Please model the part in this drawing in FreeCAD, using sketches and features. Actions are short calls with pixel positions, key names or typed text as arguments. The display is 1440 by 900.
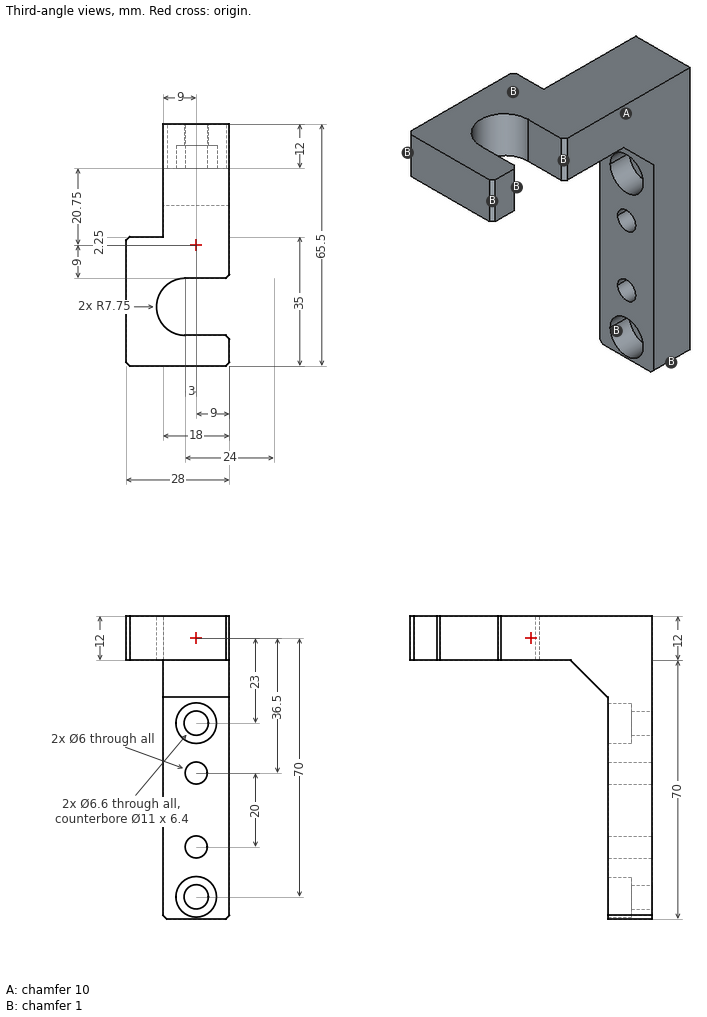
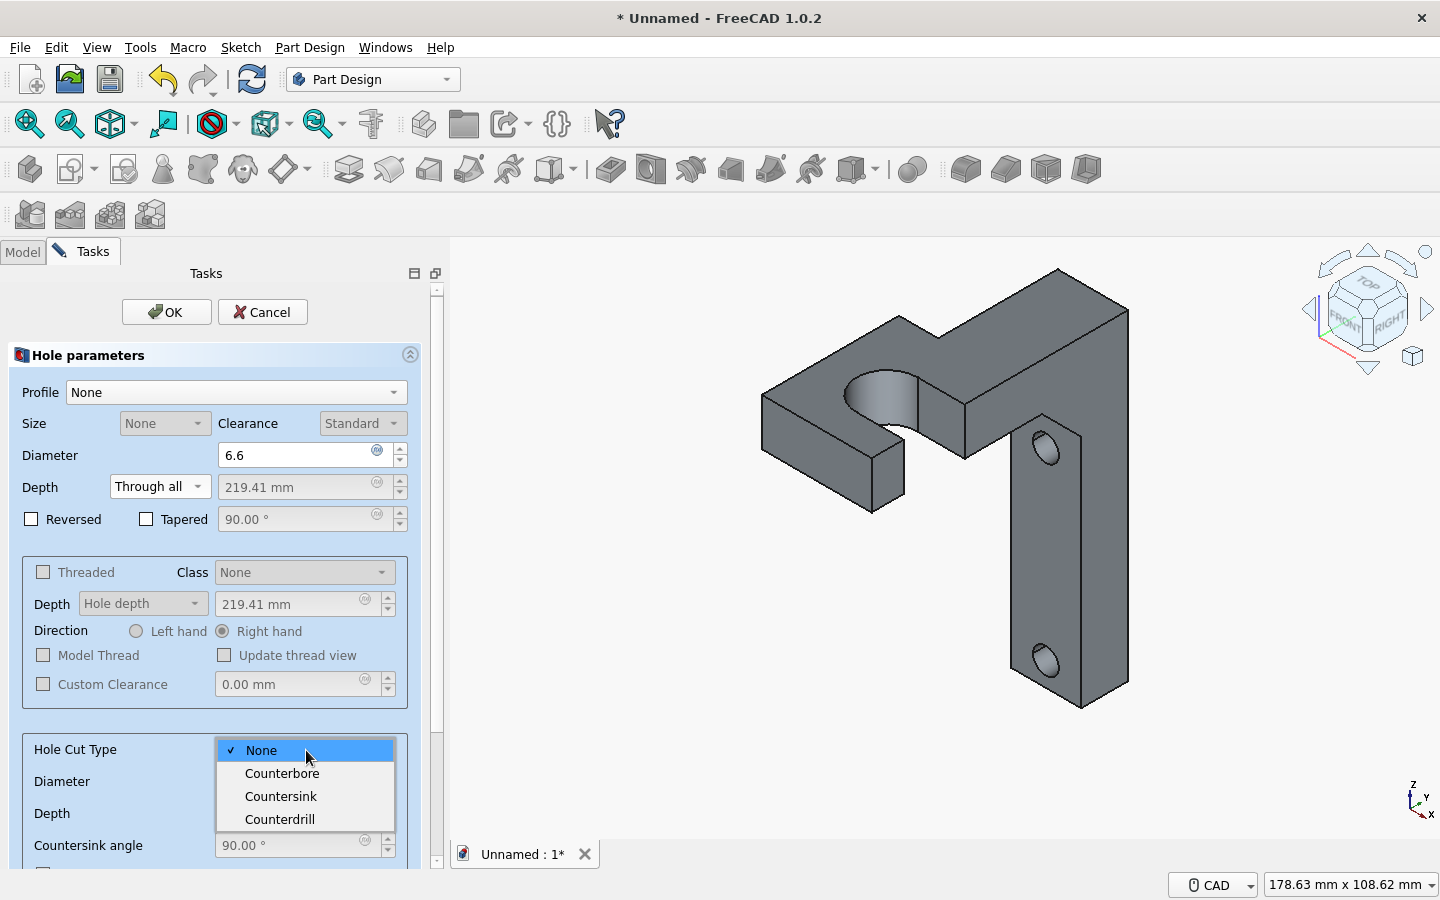
click(304, 774)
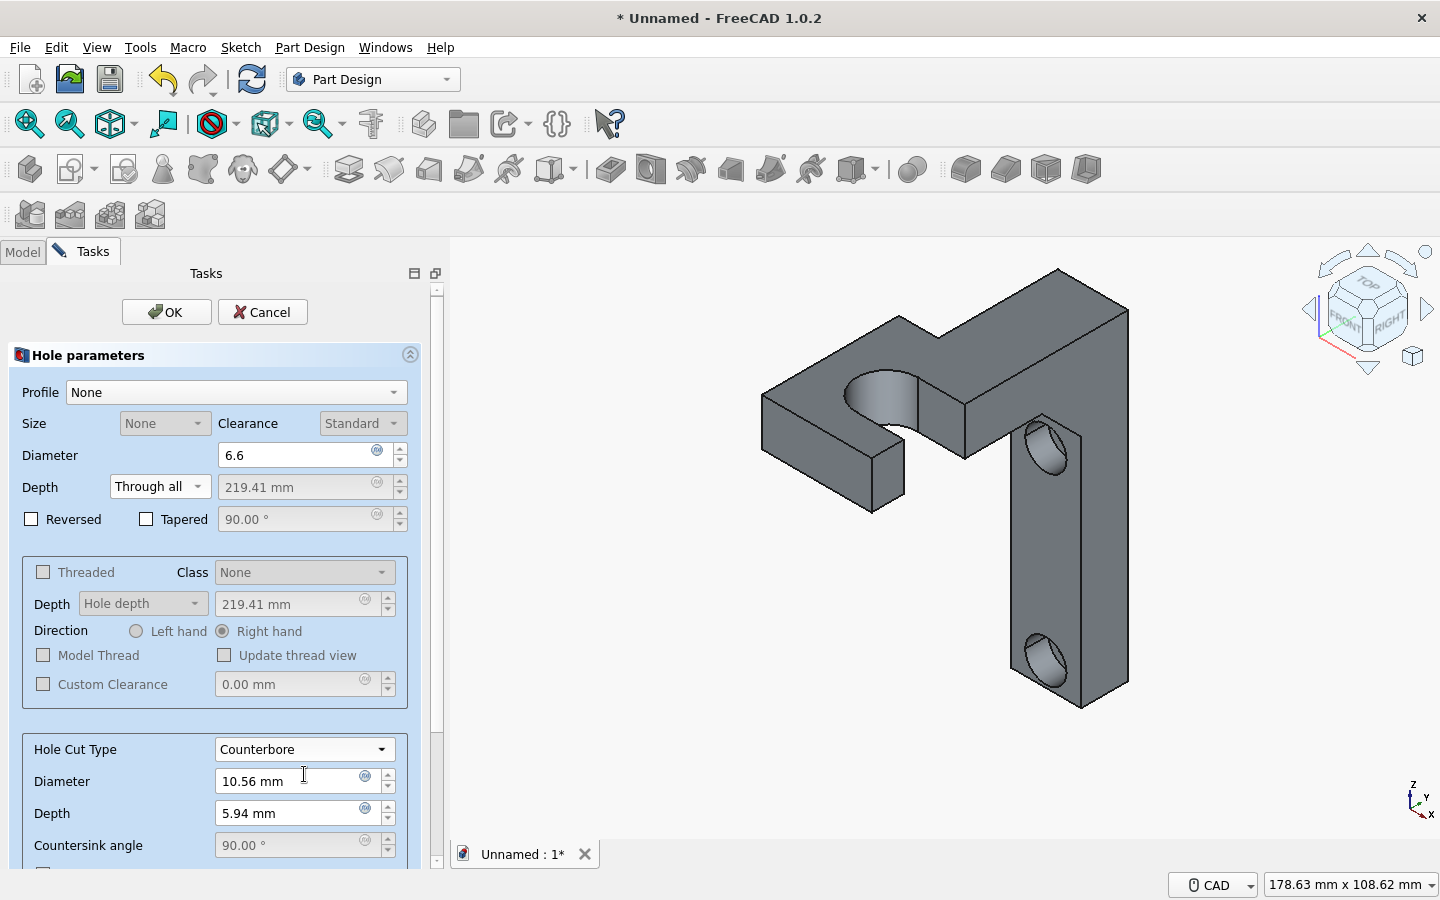
triple_click(298, 781)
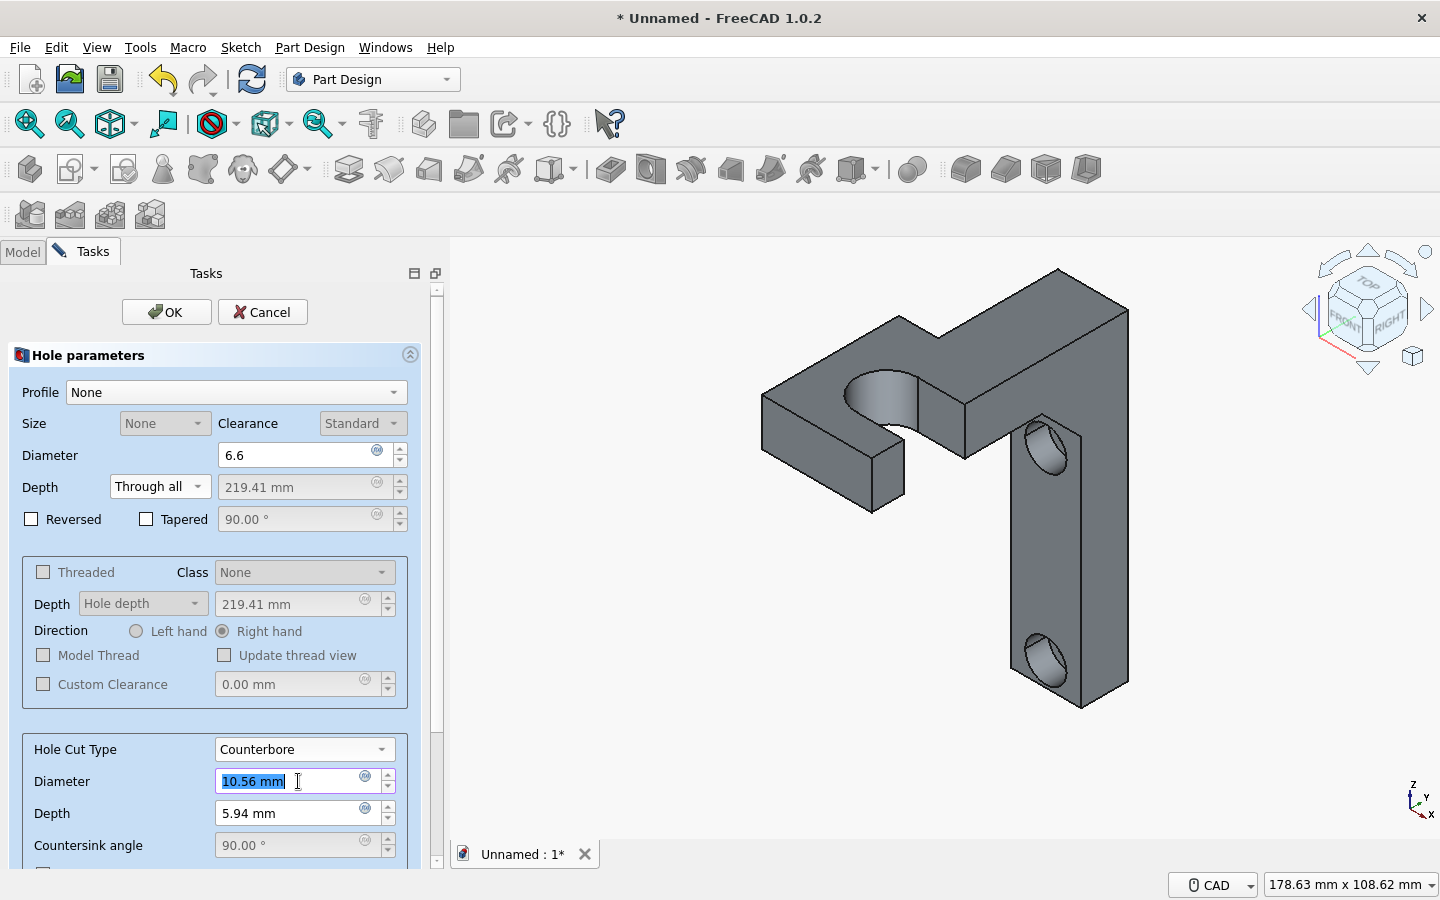
text(11)
key(Tab)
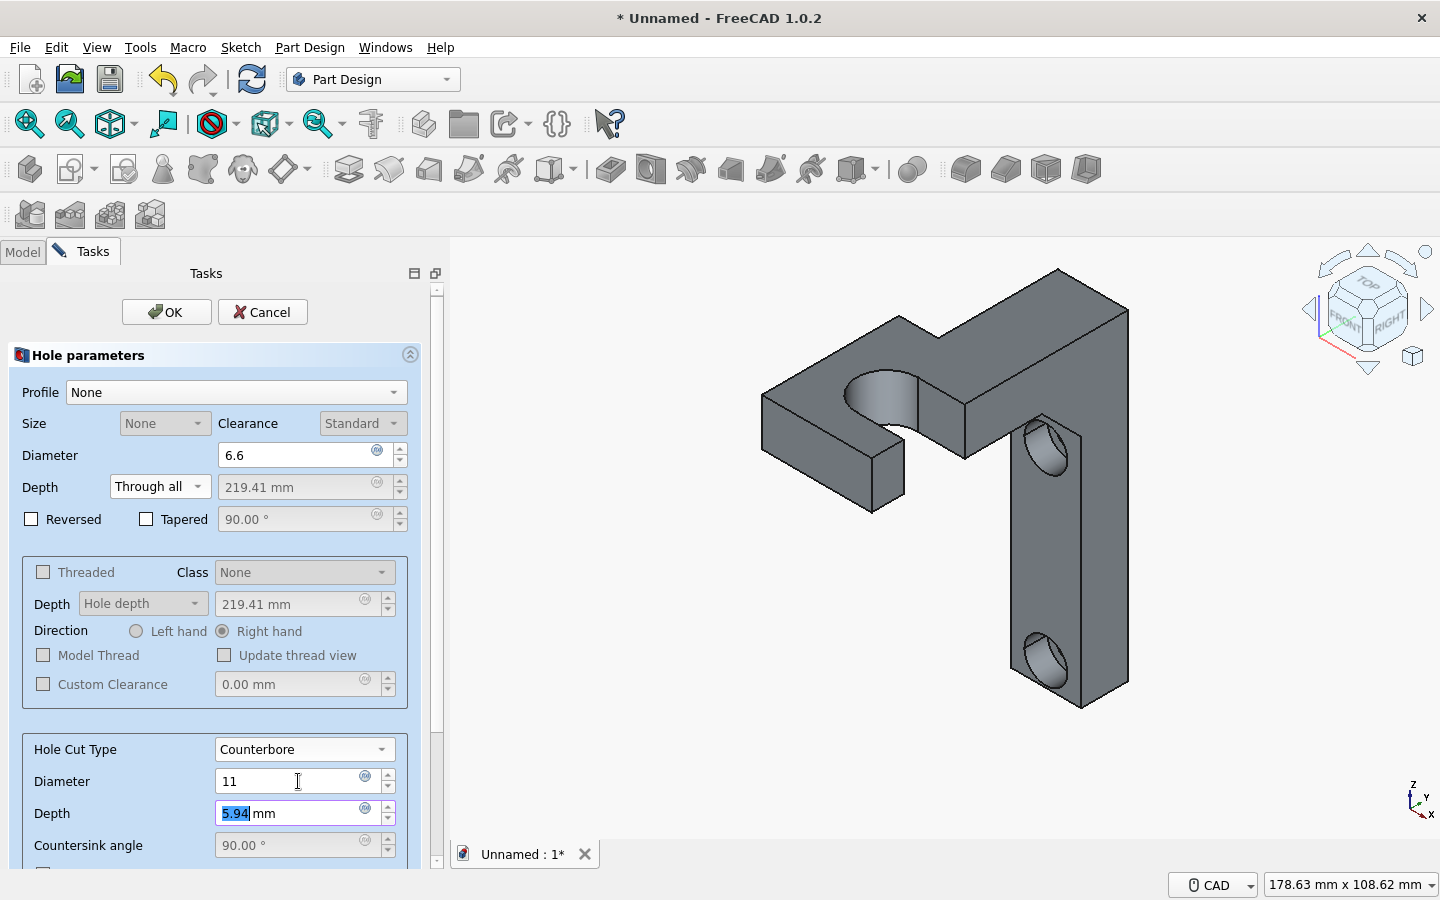
text(6.4)
key(Tab)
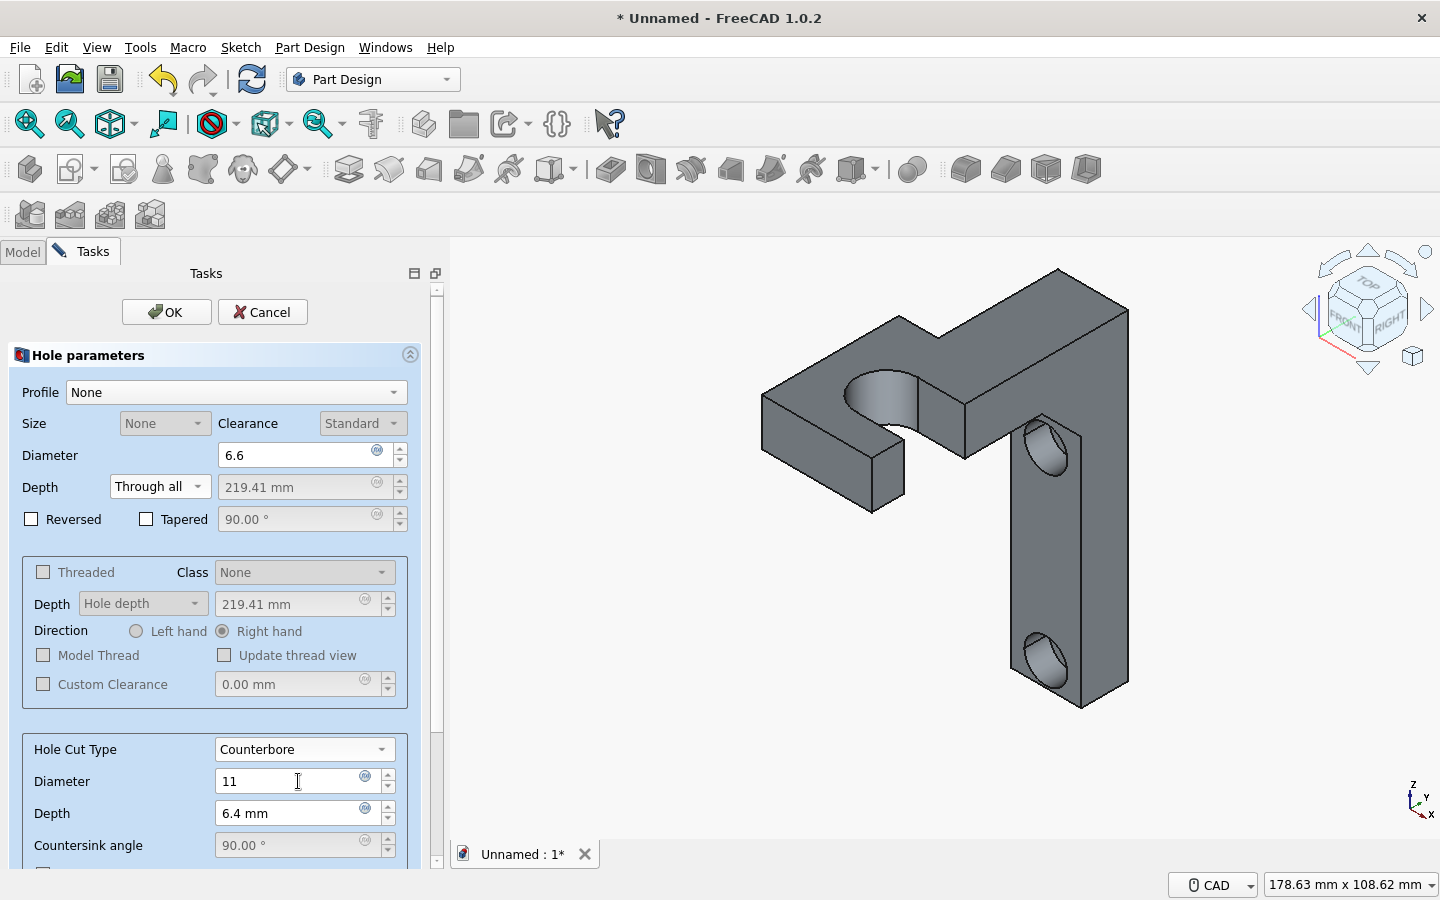
click(167, 312)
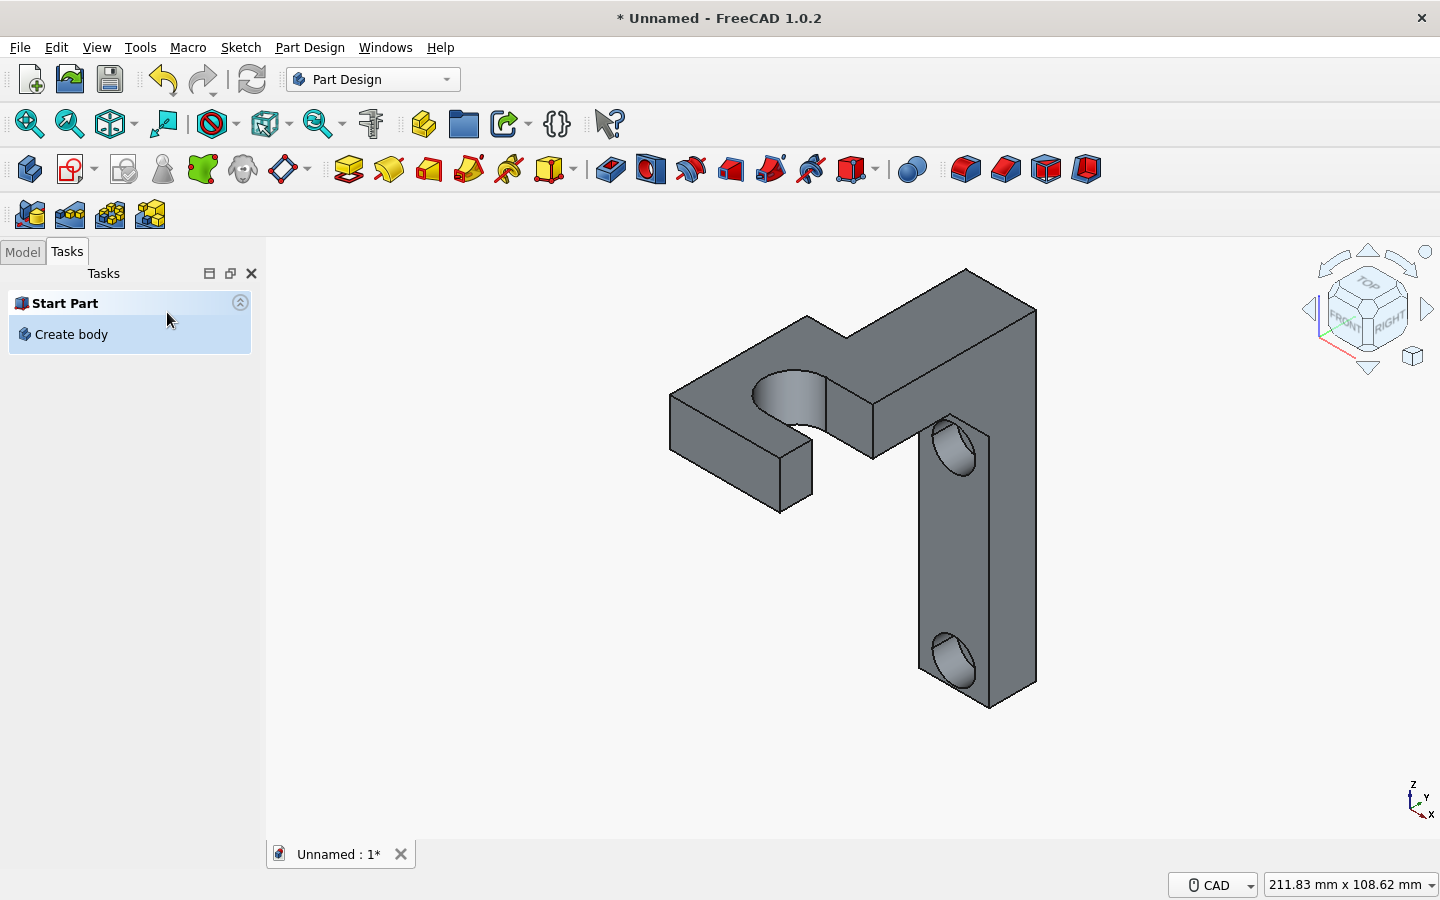
click(954, 551)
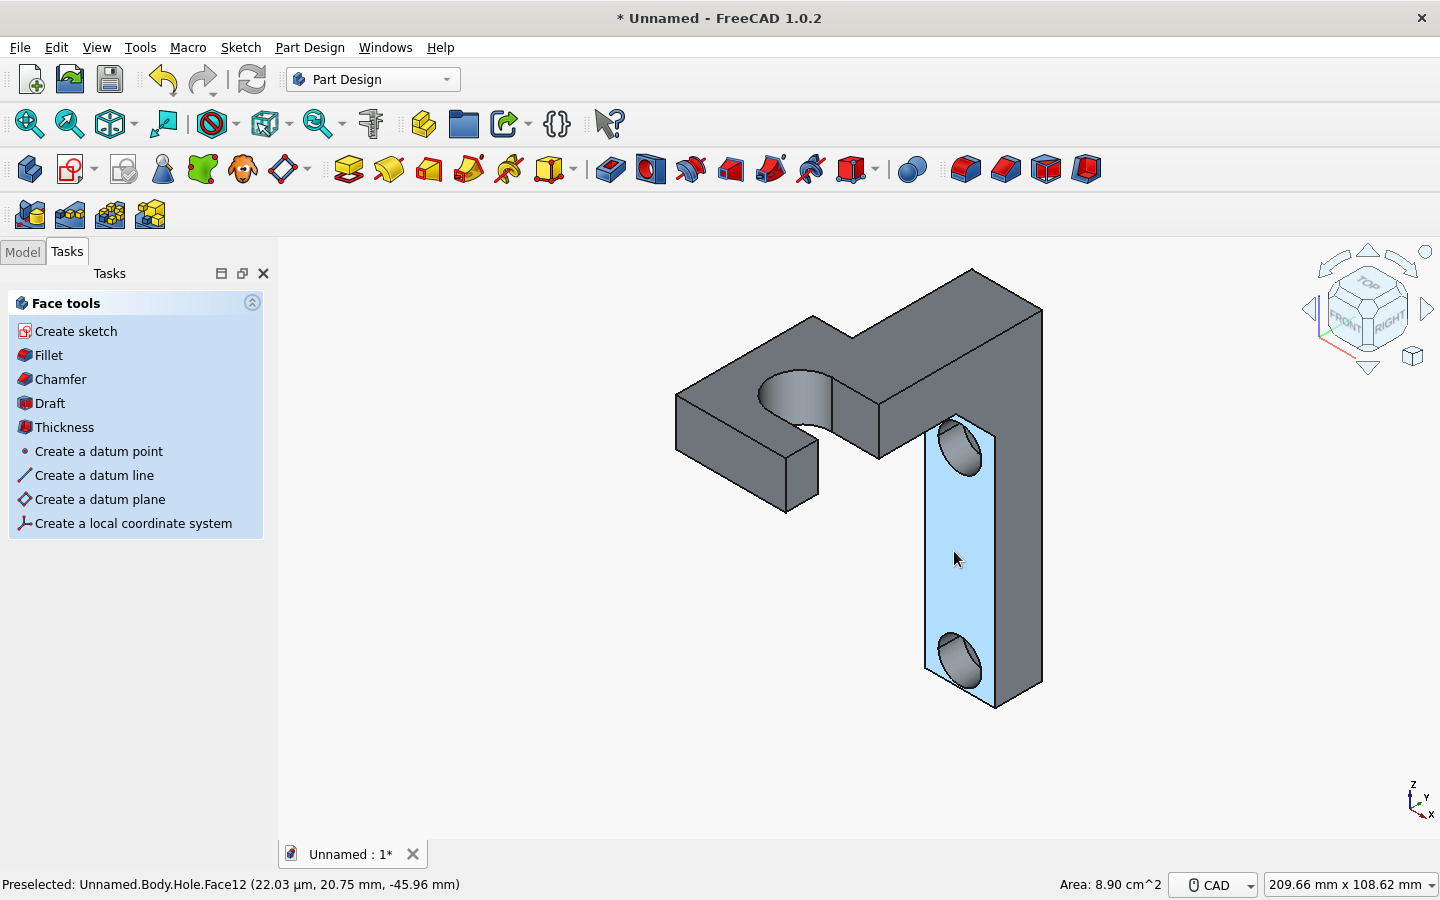
click(70, 170)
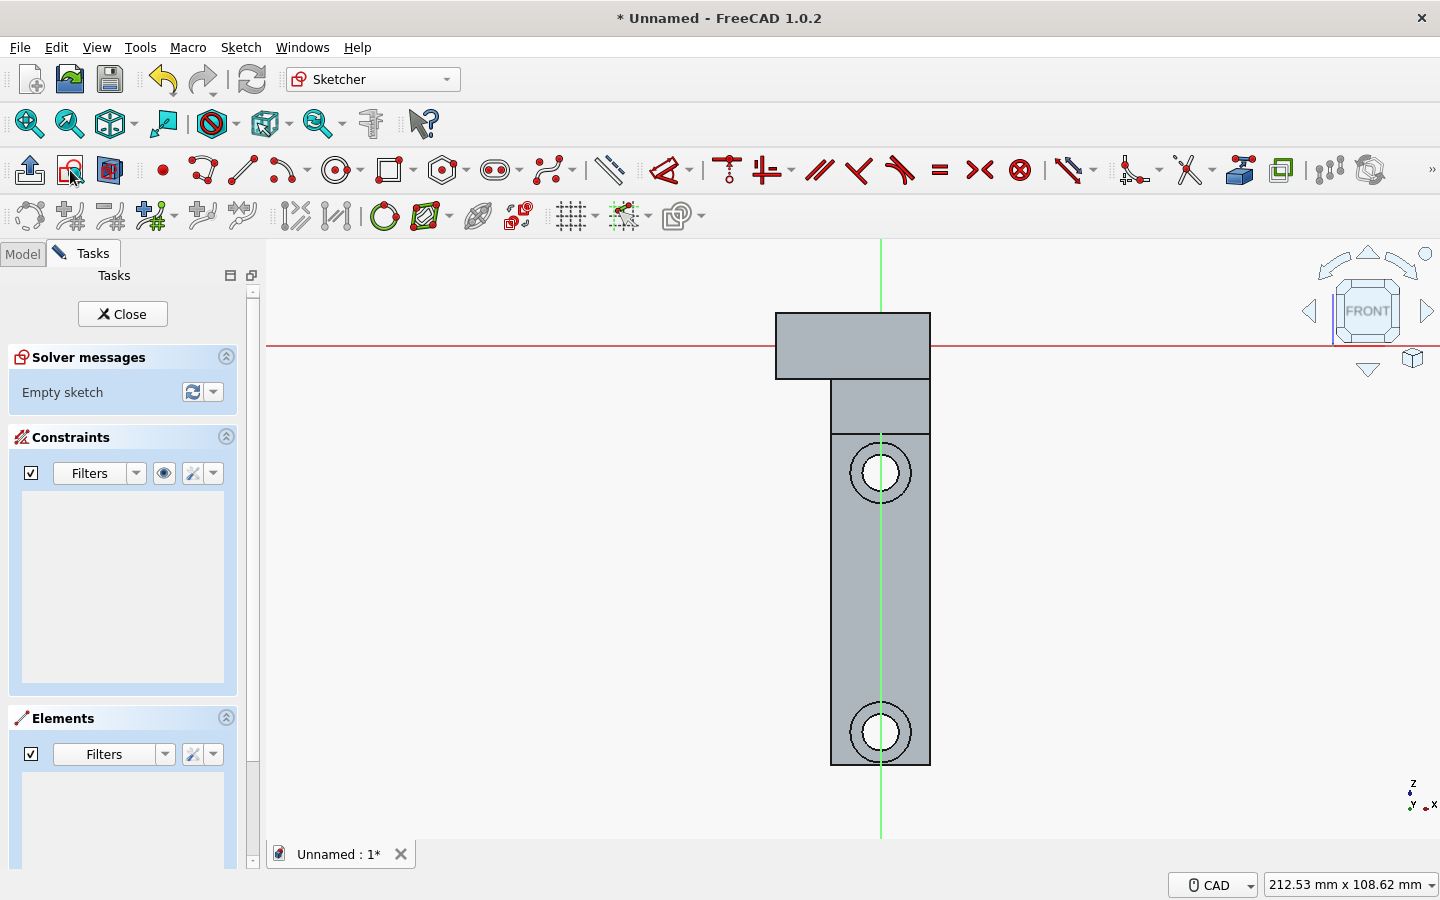
click(336, 170)